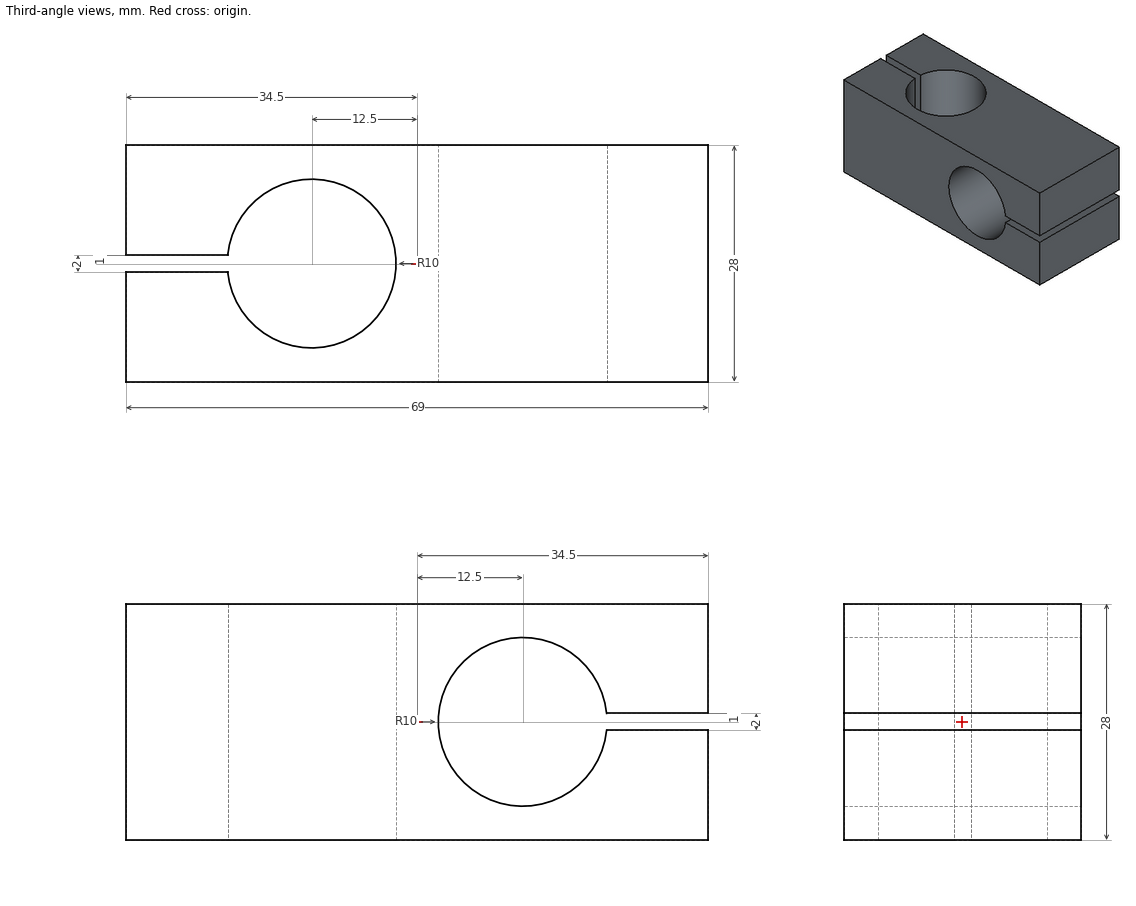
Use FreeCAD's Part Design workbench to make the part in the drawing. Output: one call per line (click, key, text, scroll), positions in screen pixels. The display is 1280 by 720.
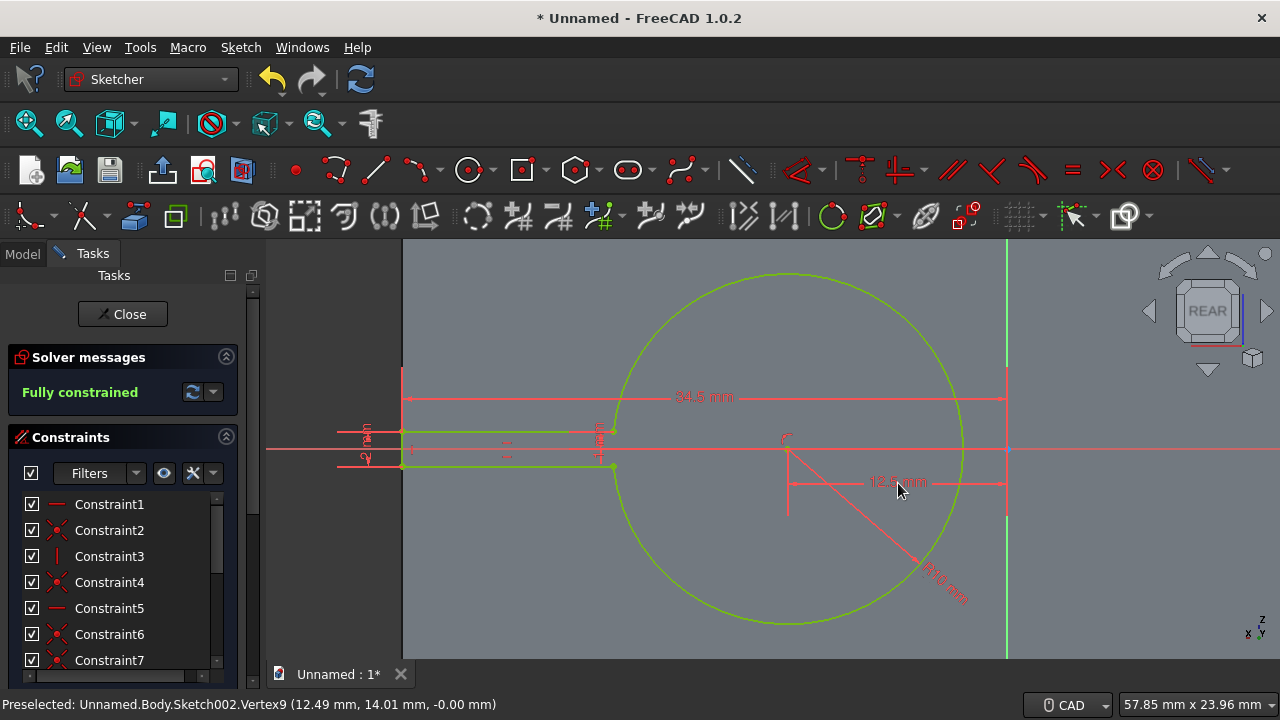
click(123, 314)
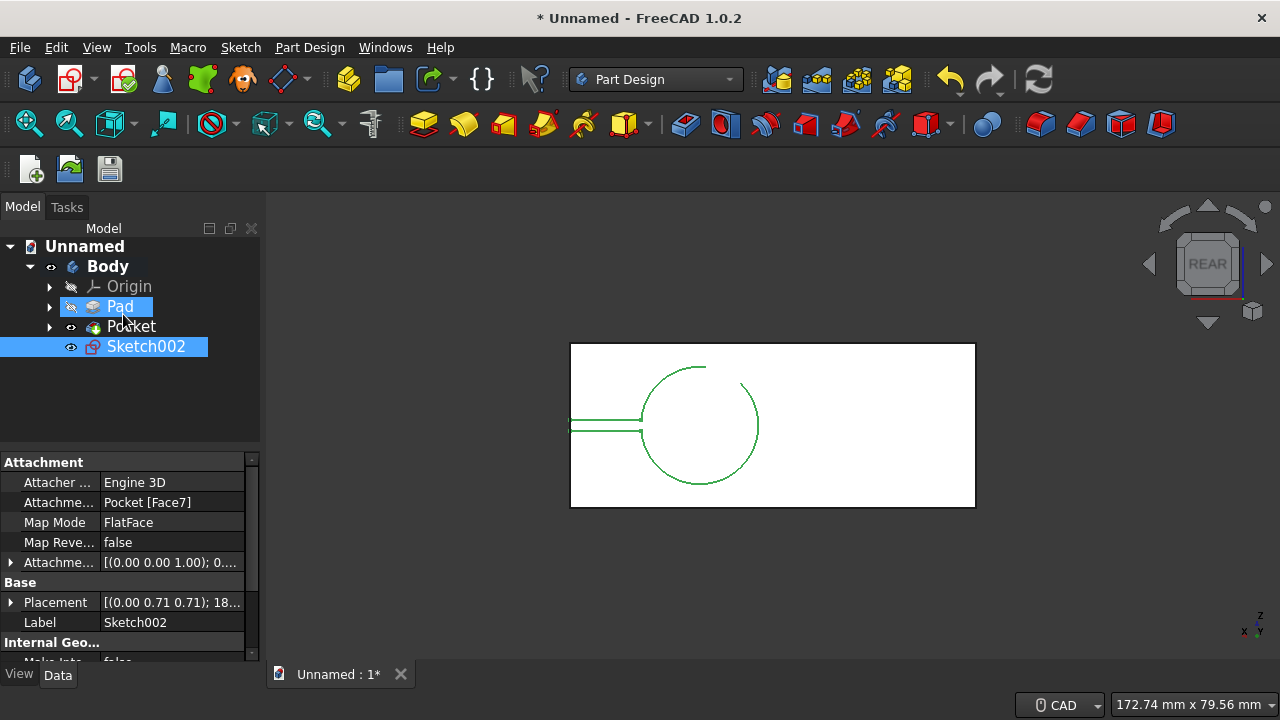
click(686, 124)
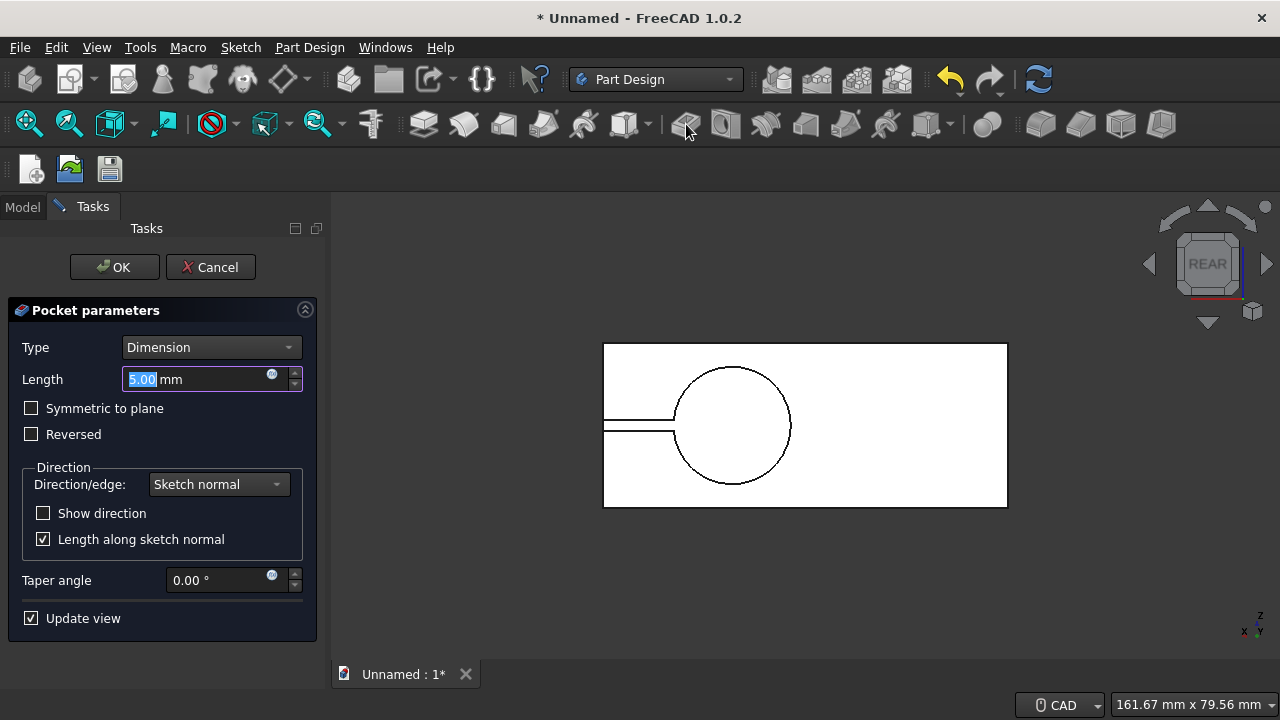
click(212, 348)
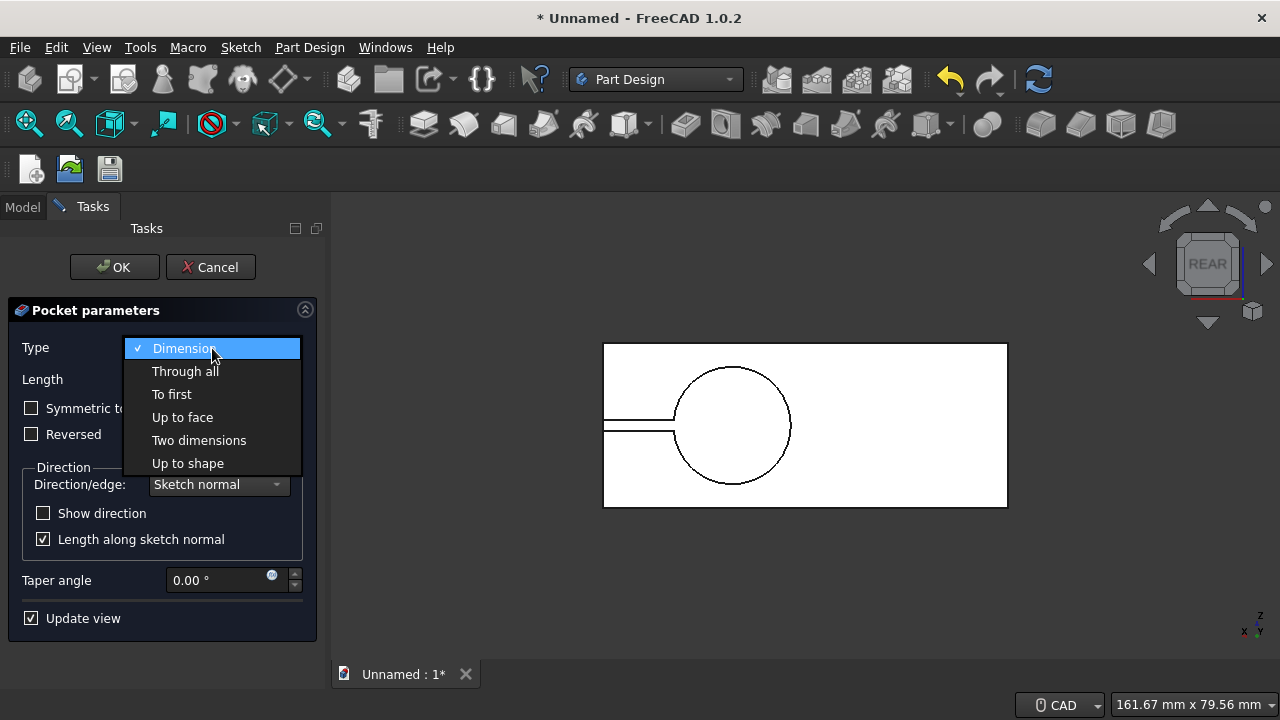
click(212, 372)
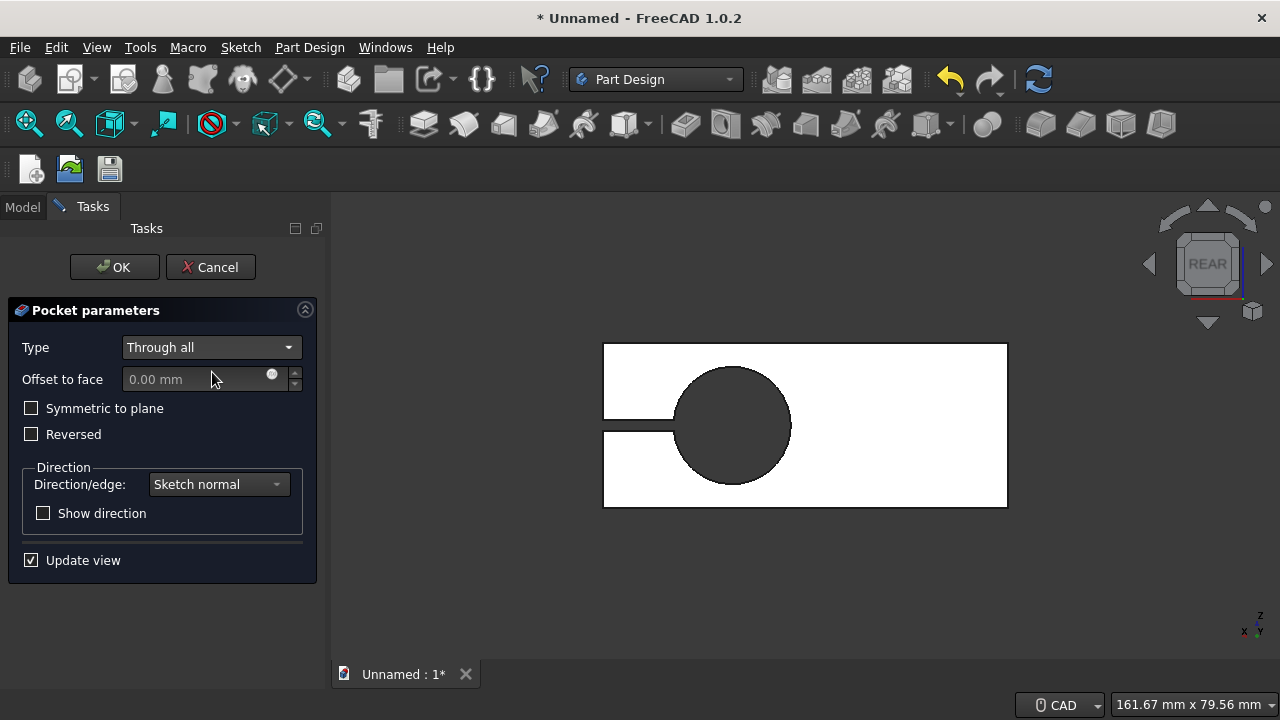
click(115, 267)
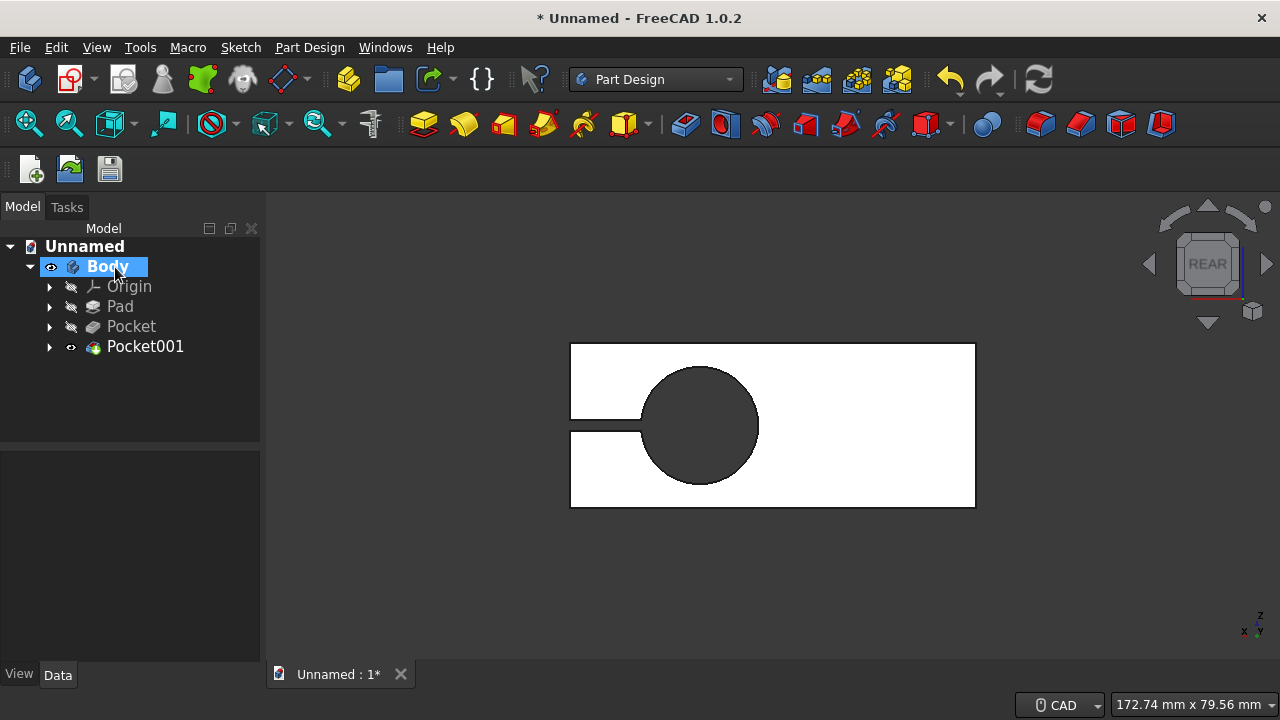
key(0)